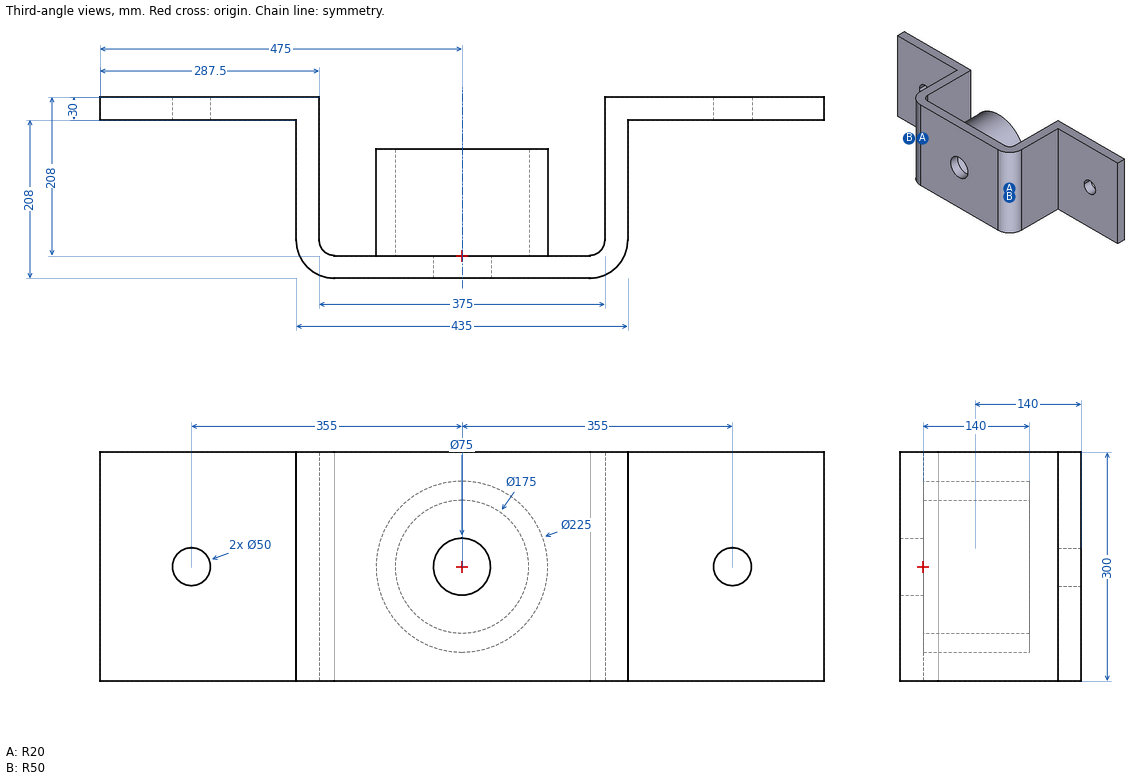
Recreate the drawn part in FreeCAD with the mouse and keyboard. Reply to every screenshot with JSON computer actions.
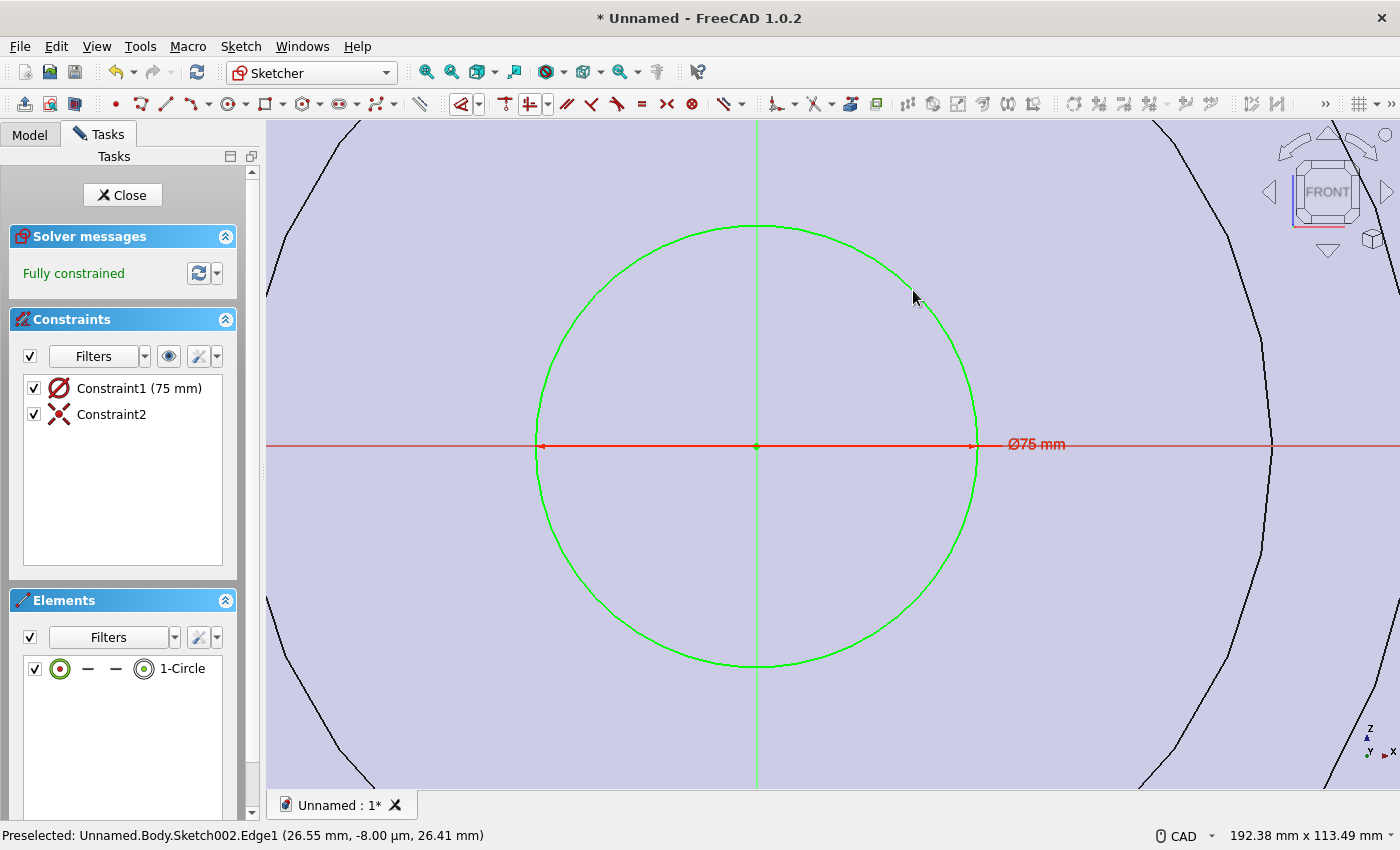
{"action": "left_click", "coordinate": [123, 195]}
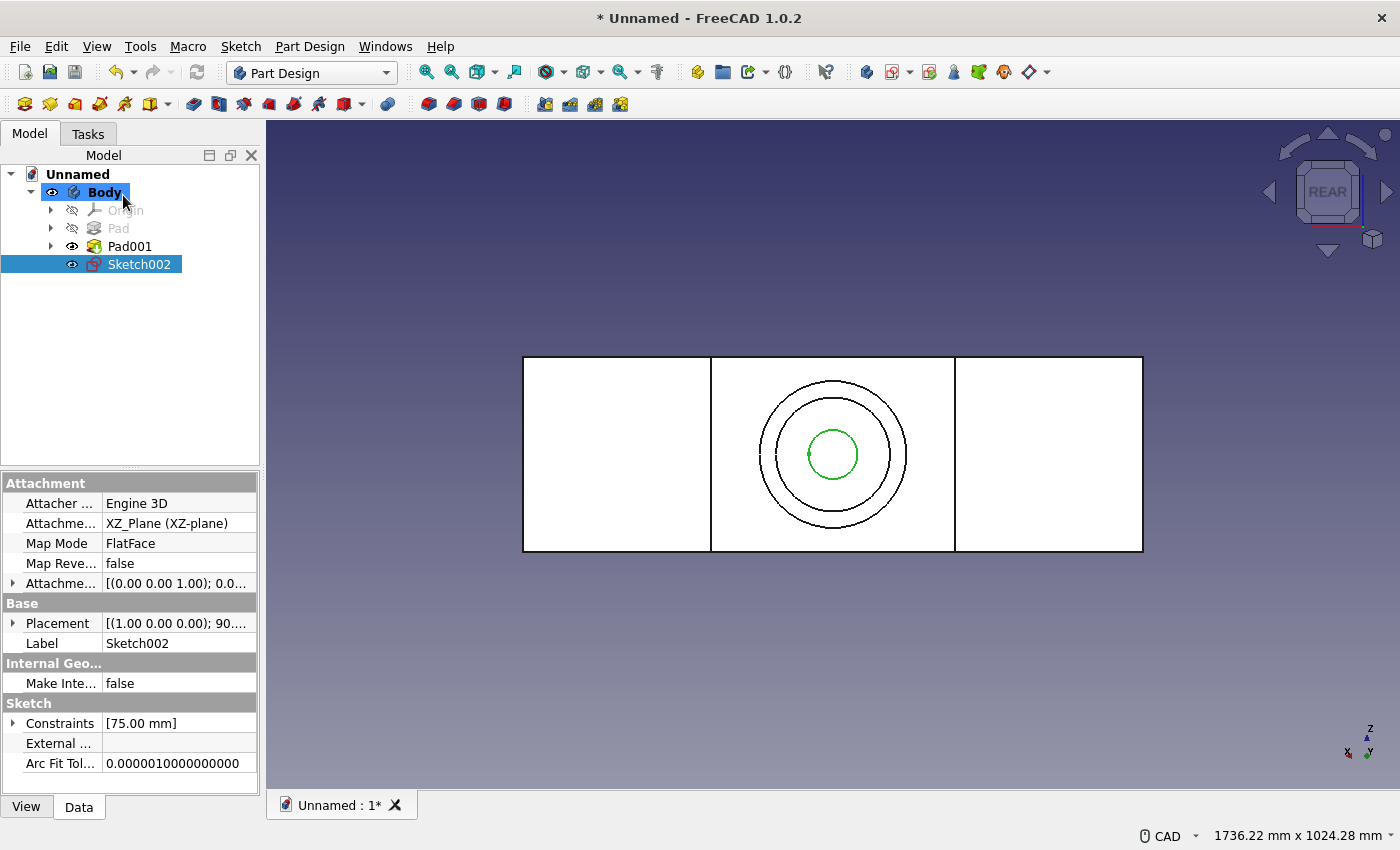
{"action": "left_click", "coordinate": [194, 104]}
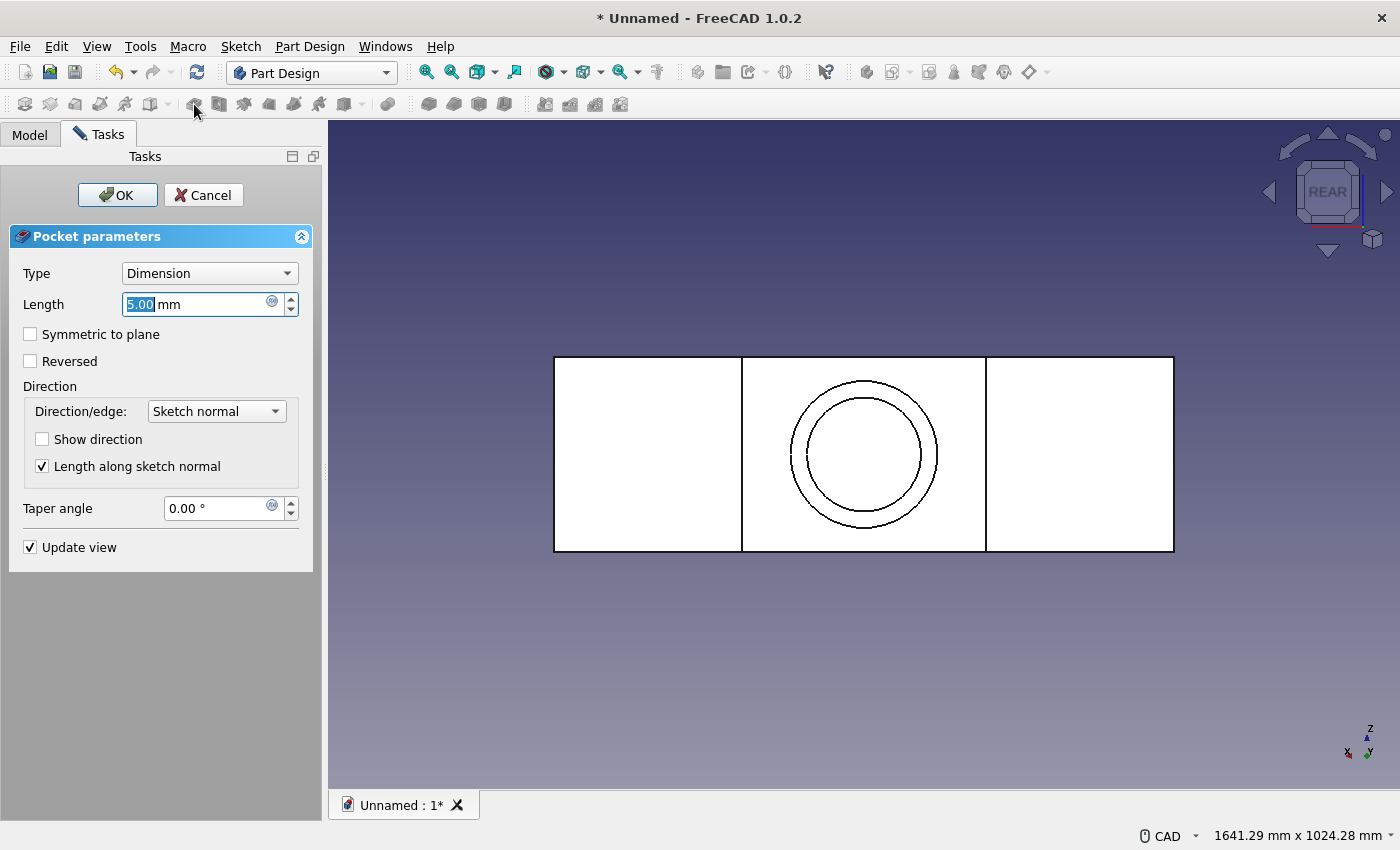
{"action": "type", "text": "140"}
{"action": "key", "text": "Tab"}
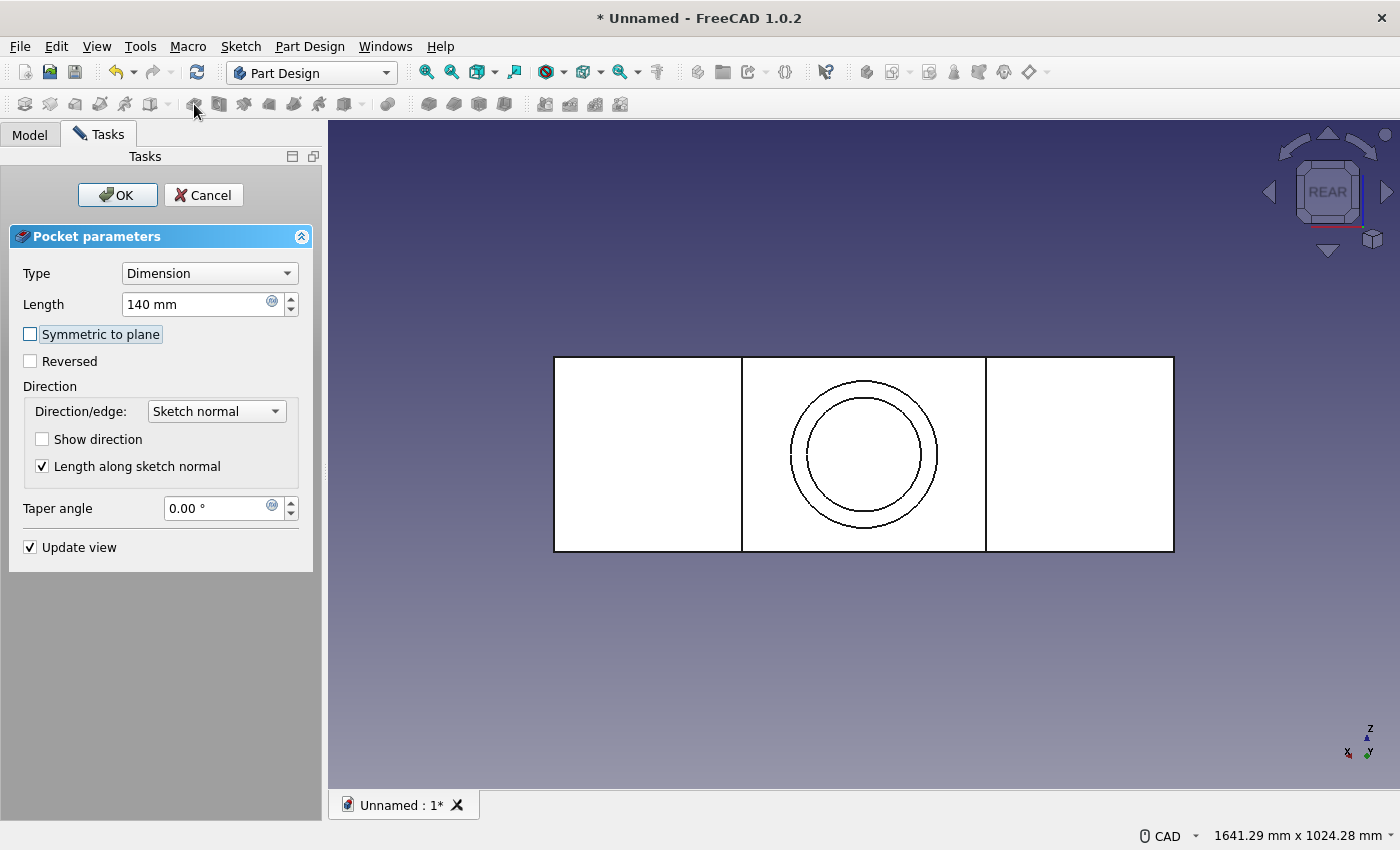
{"action": "left_click", "coordinate": [31, 361]}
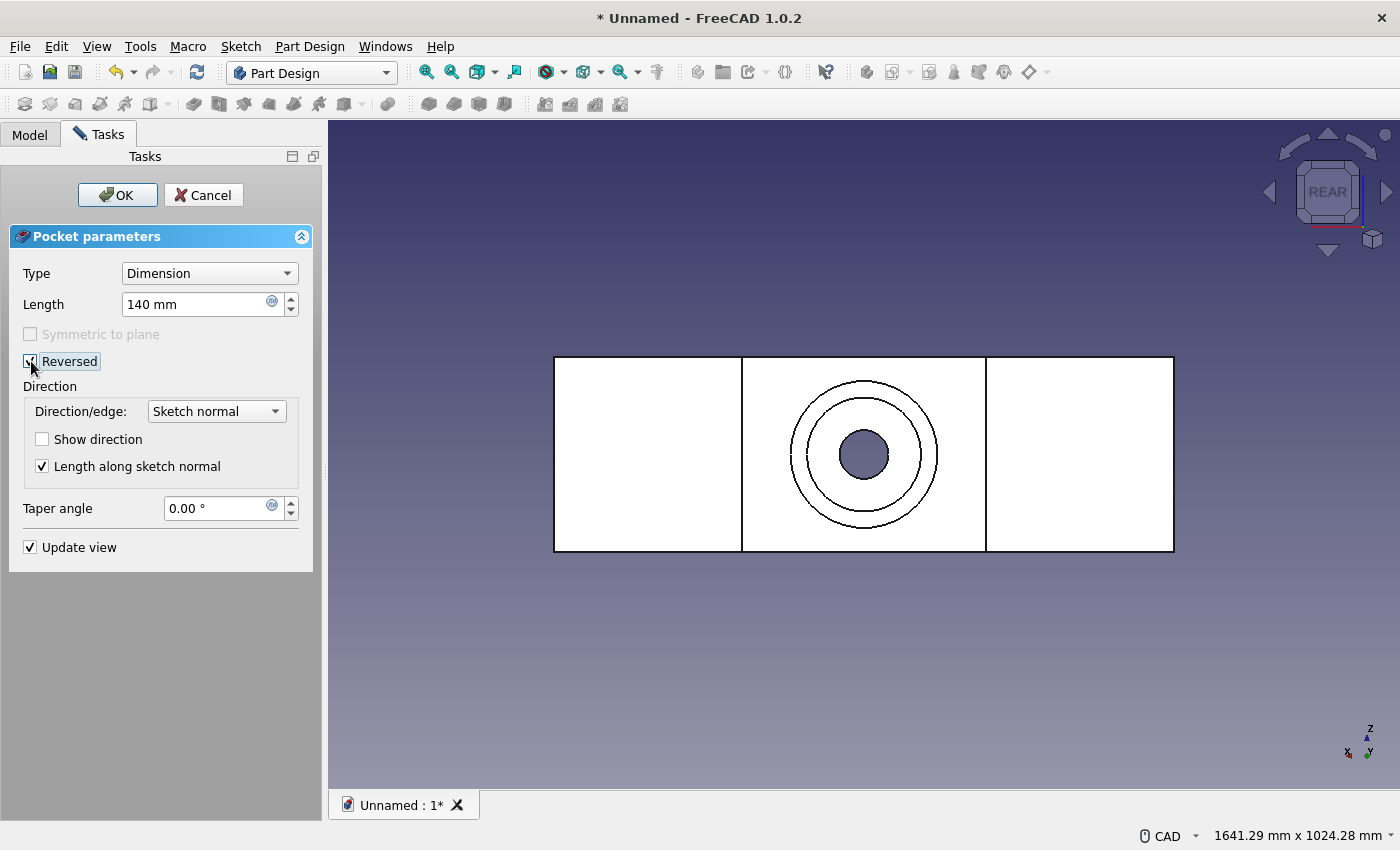
{"action": "left_click", "coordinate": [118, 195]}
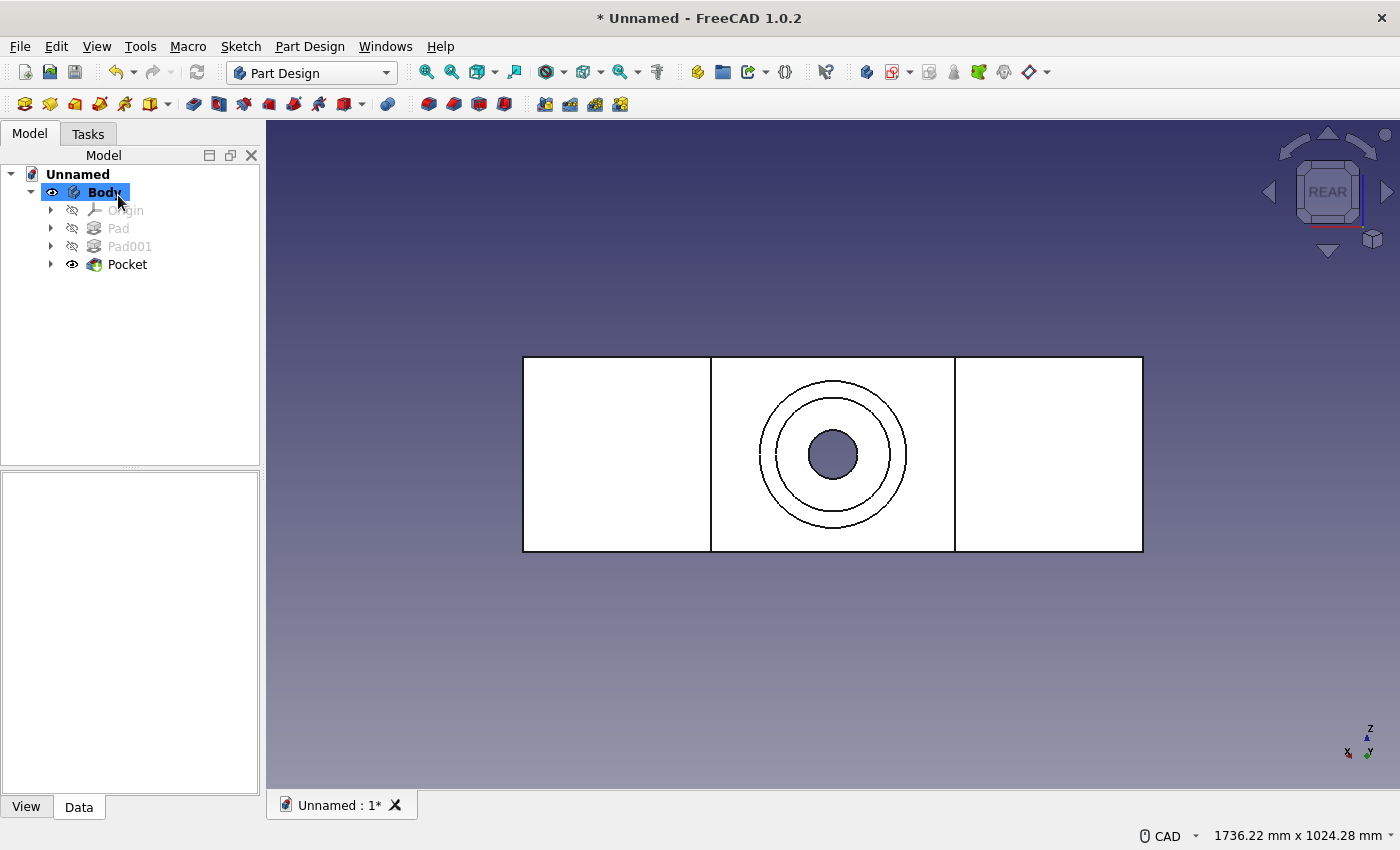
{"action": "left_click", "coordinate": [1049, 454]}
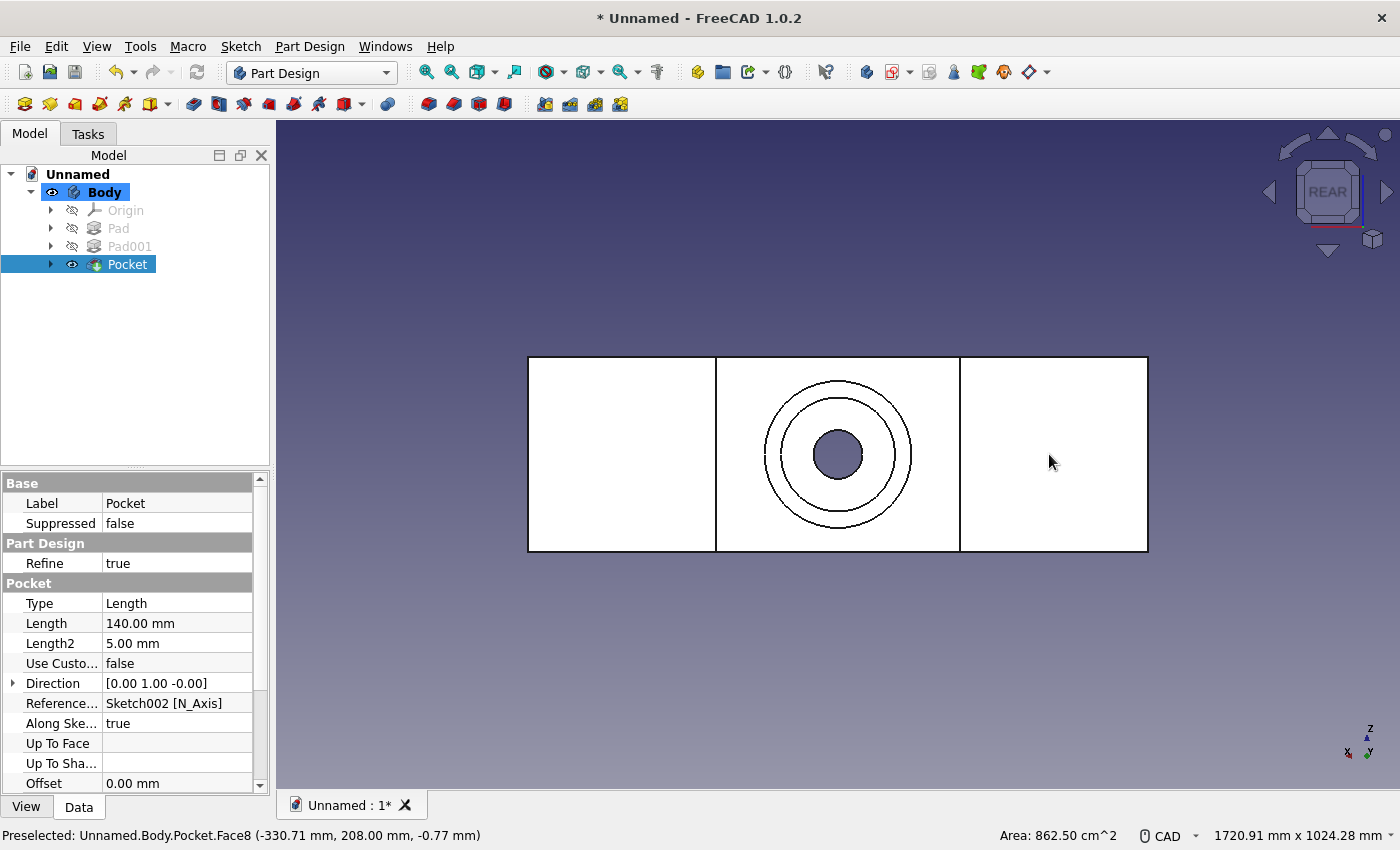
{"action": "left_click", "coordinate": [892, 72]}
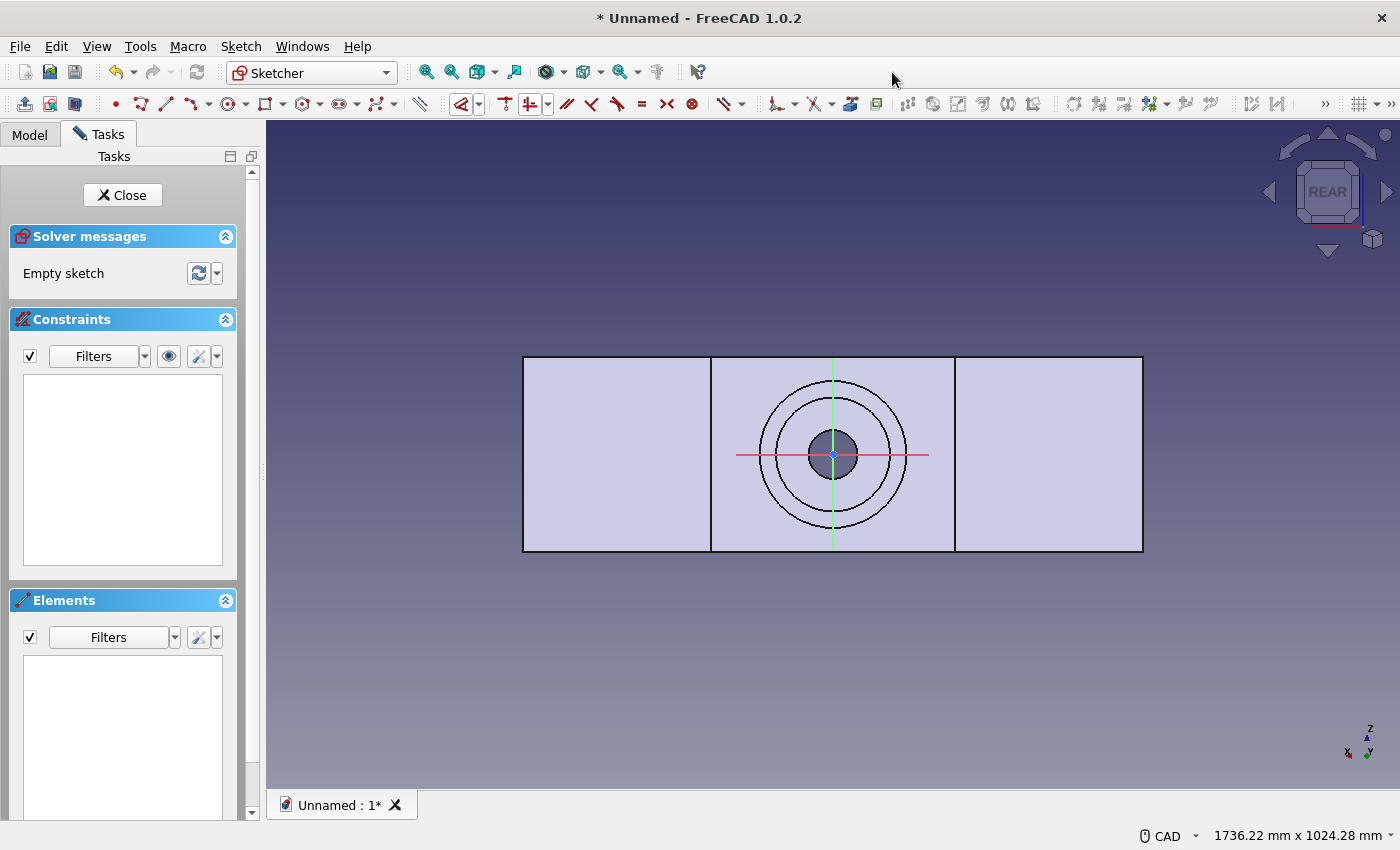
{"action": "left_click", "coordinate": [228, 104]}